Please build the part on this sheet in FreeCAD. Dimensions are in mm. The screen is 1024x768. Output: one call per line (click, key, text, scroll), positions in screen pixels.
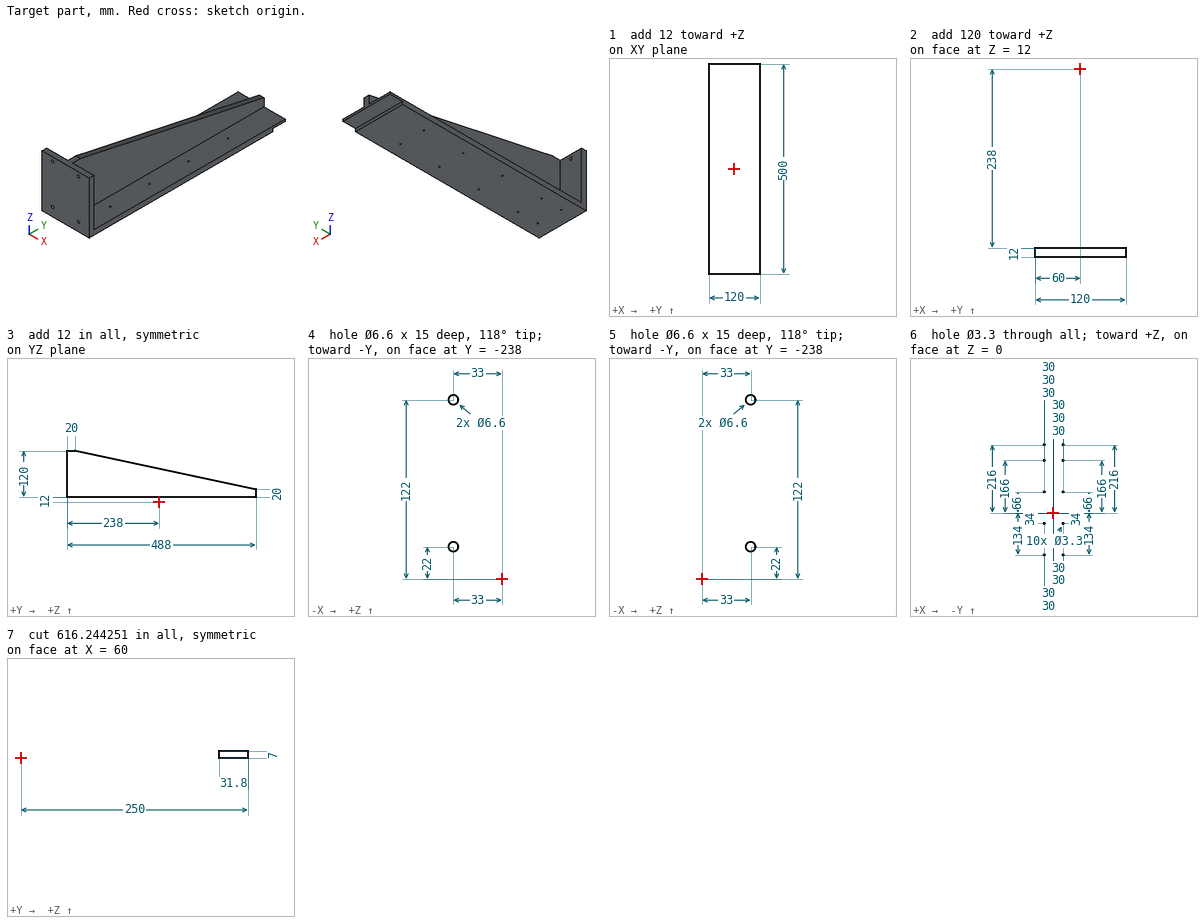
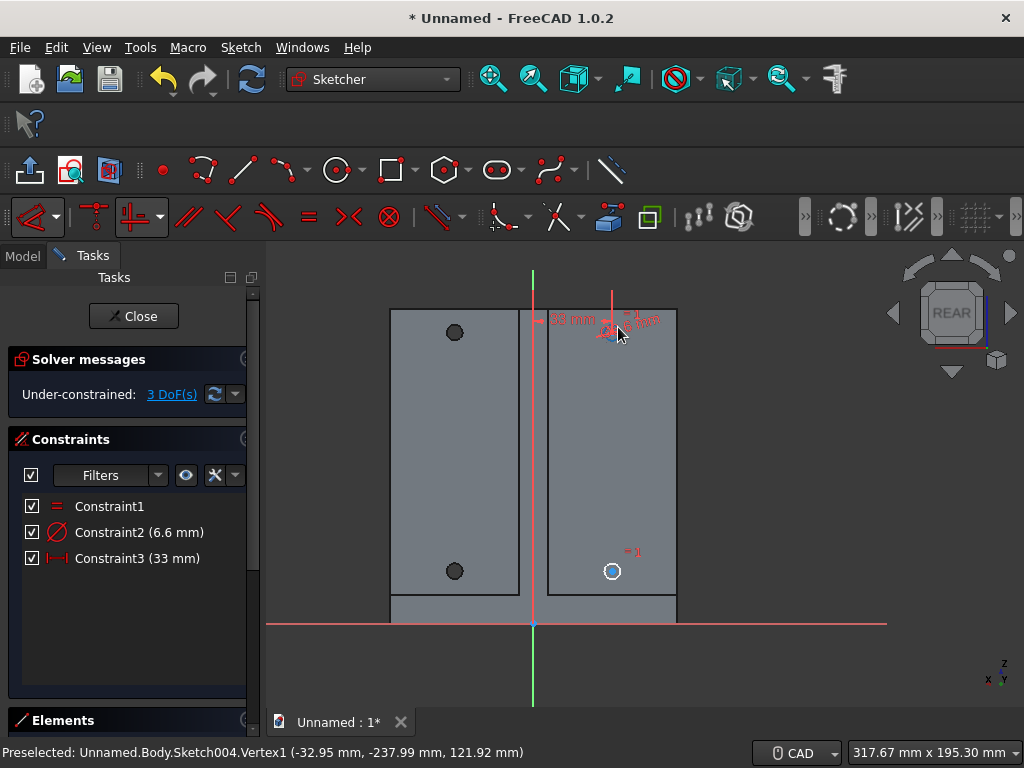
click(612, 571)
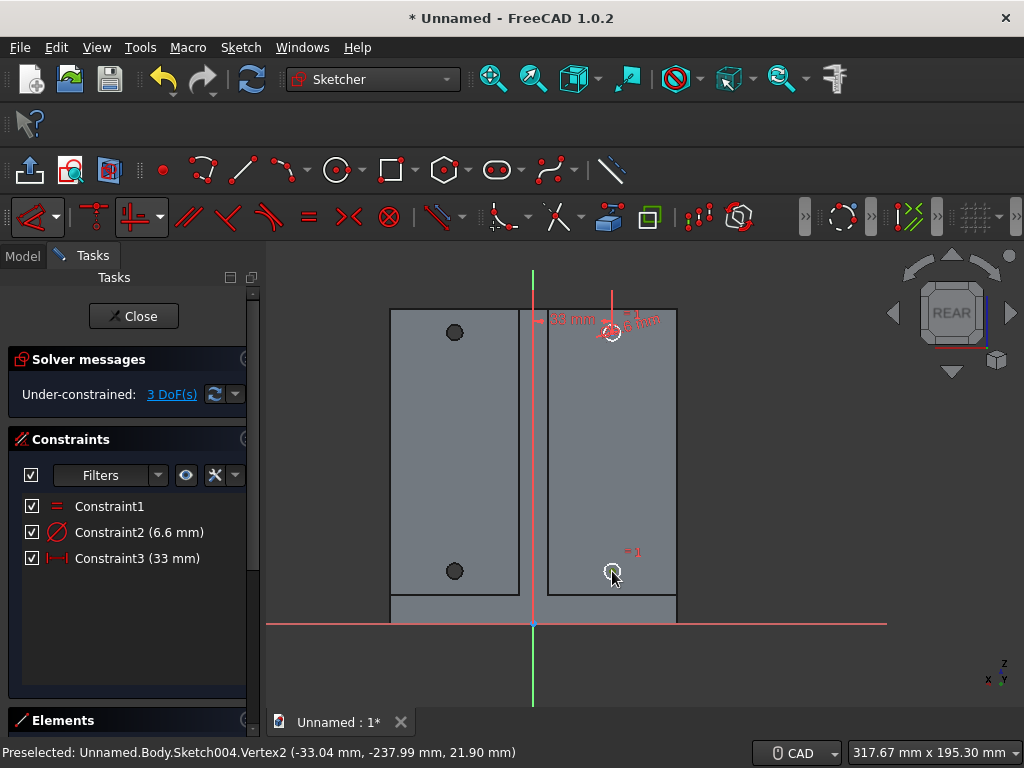
click(58, 218)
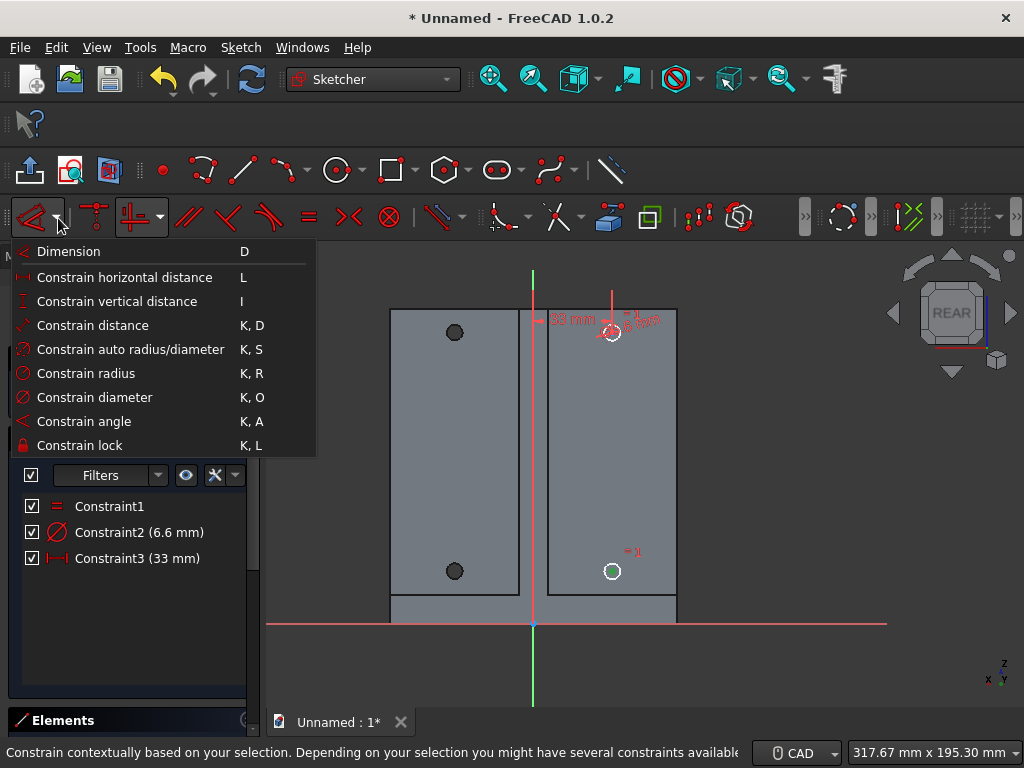
click(164, 277)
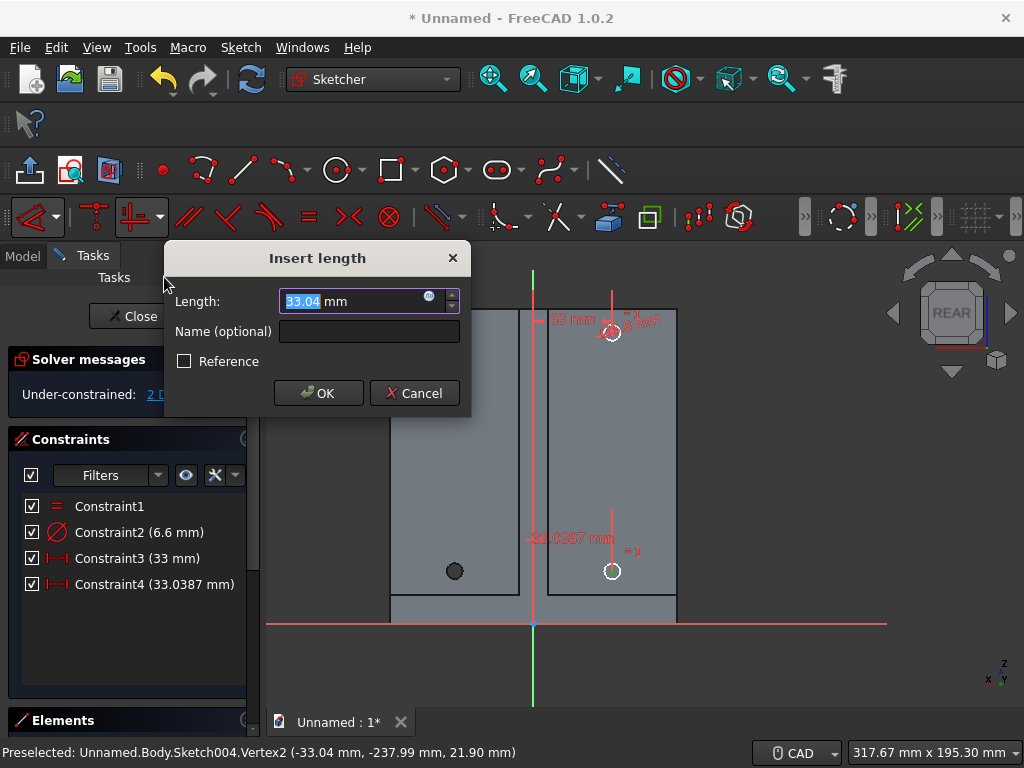
text(33)
key(Return)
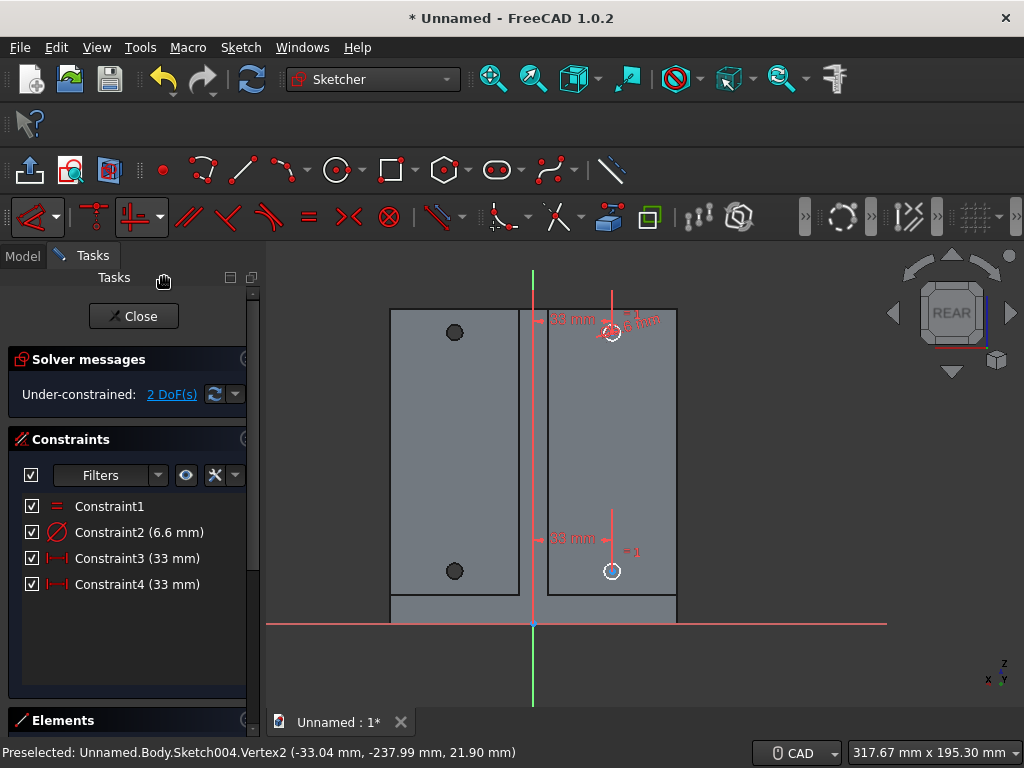
click(612, 571)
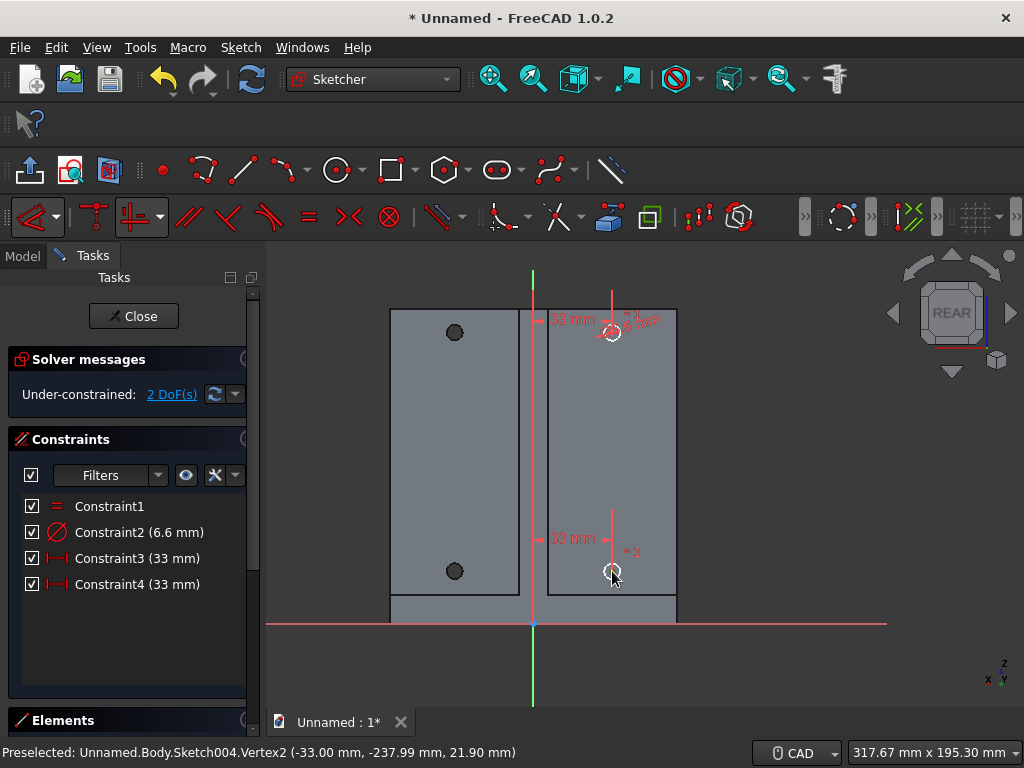
click(58, 218)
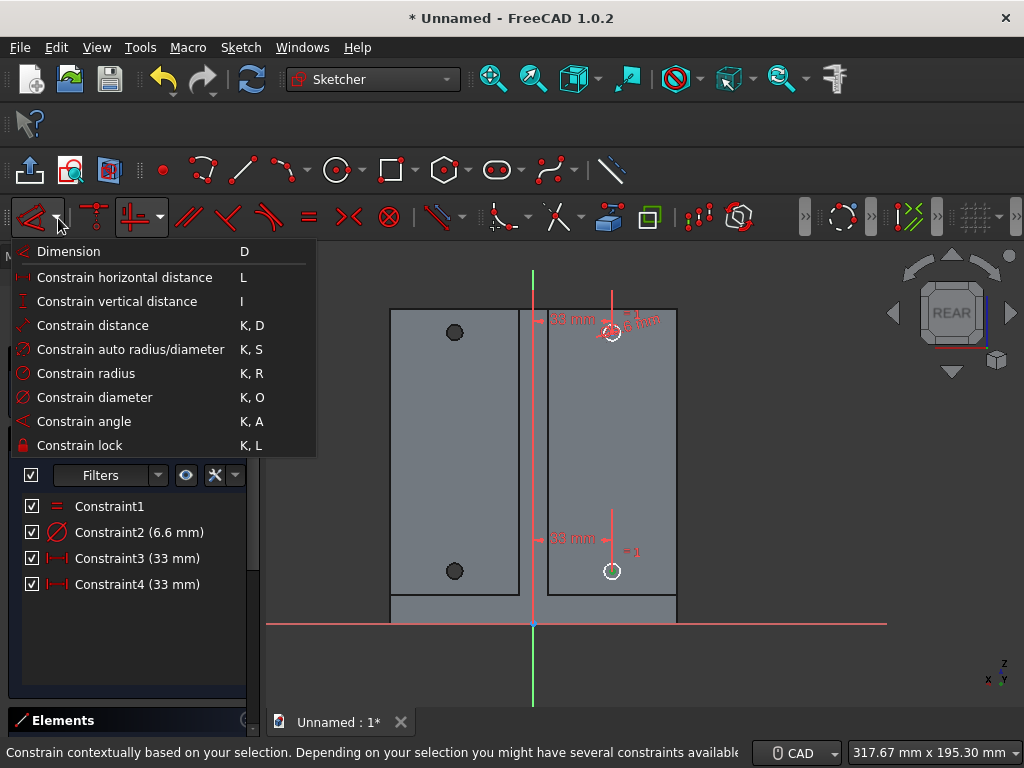
click(164, 301)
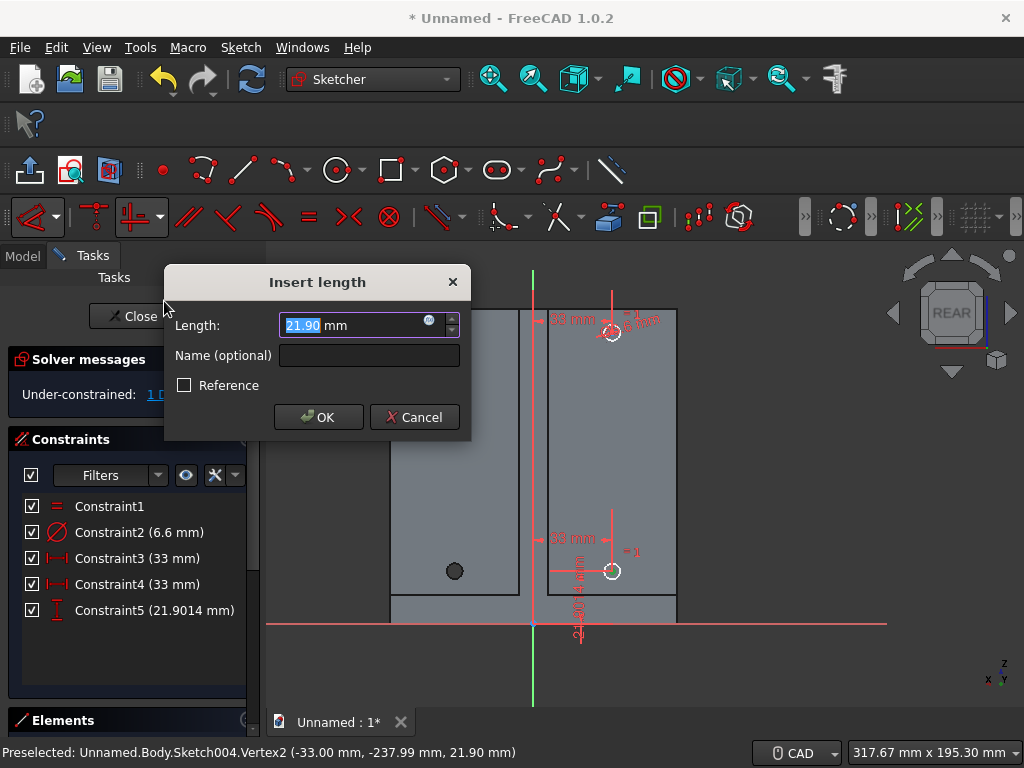
text(22)
key(Return)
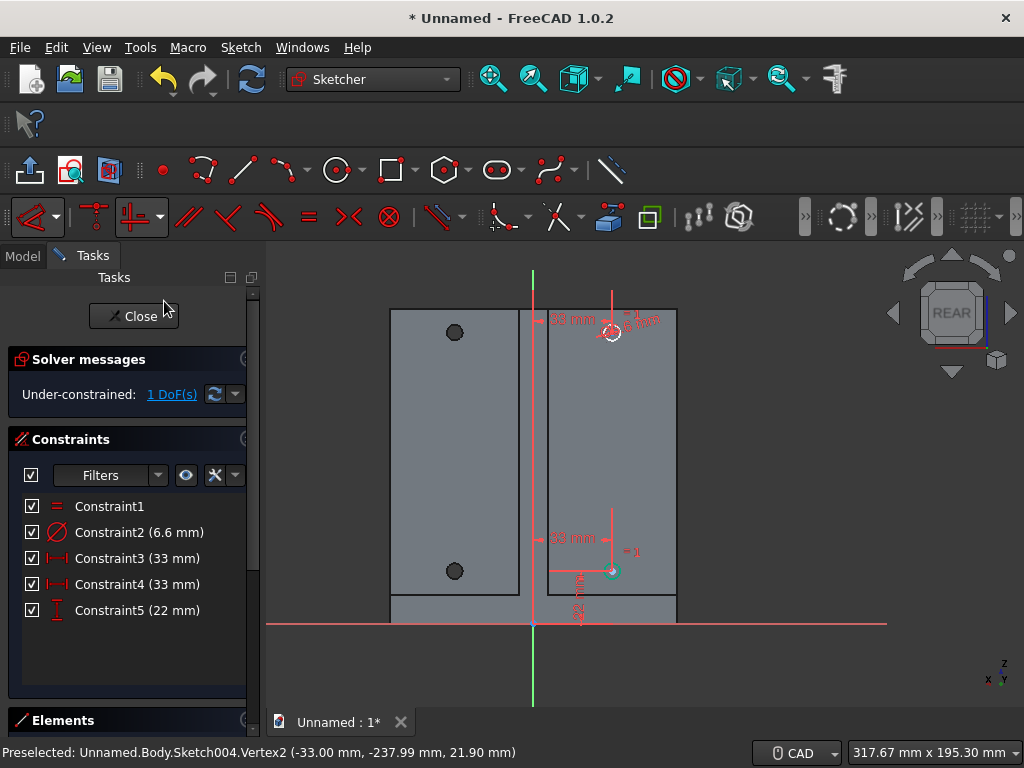
click(612, 333)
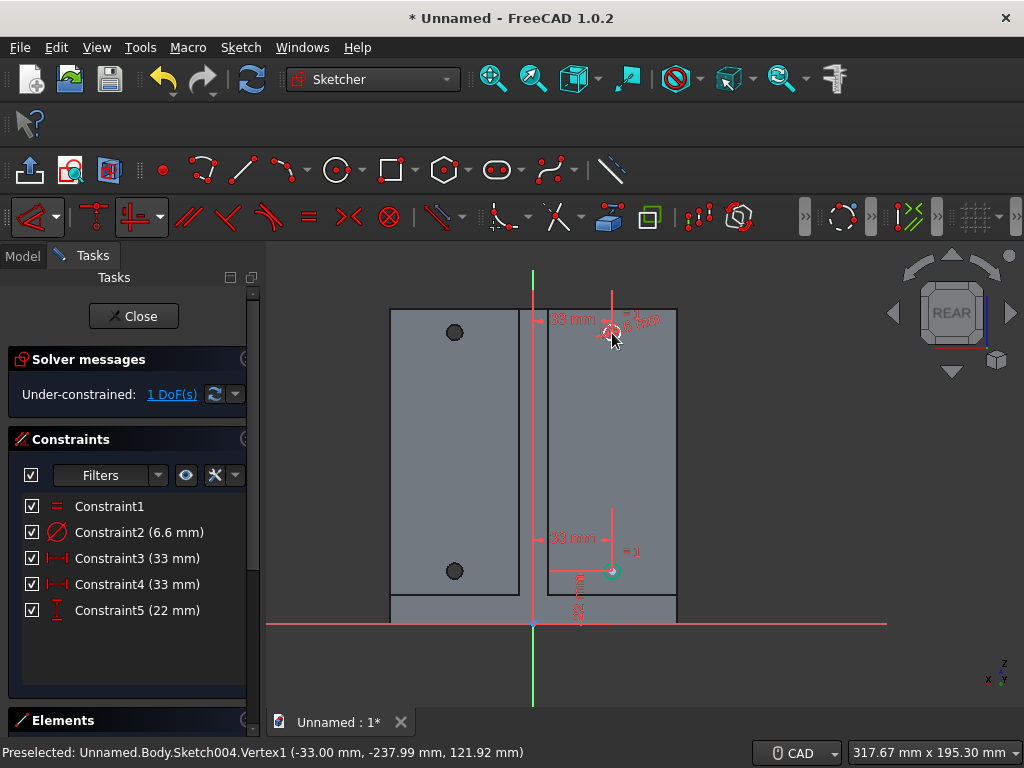
click(58, 218)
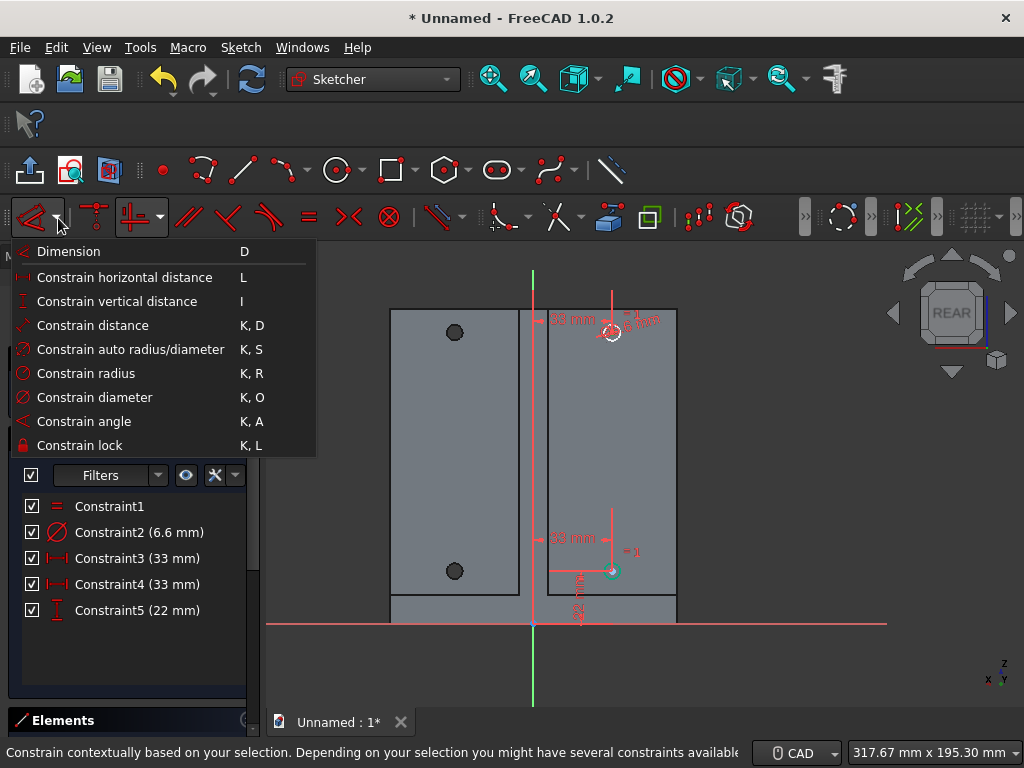
click(164, 301)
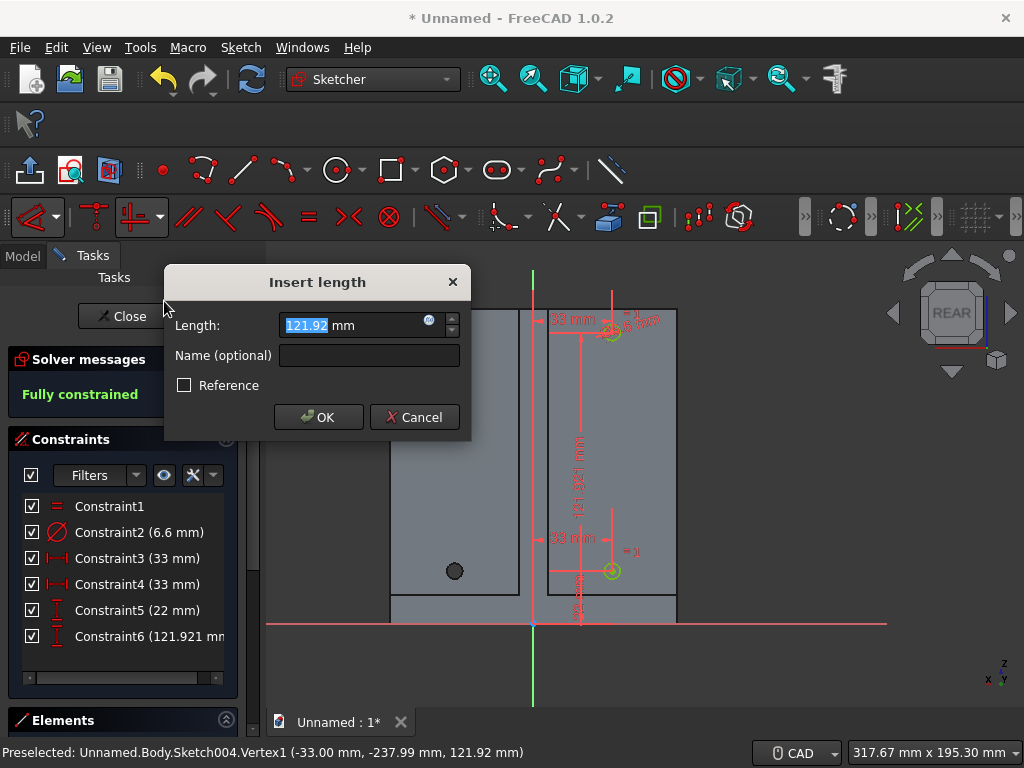
text(122)
key(Return)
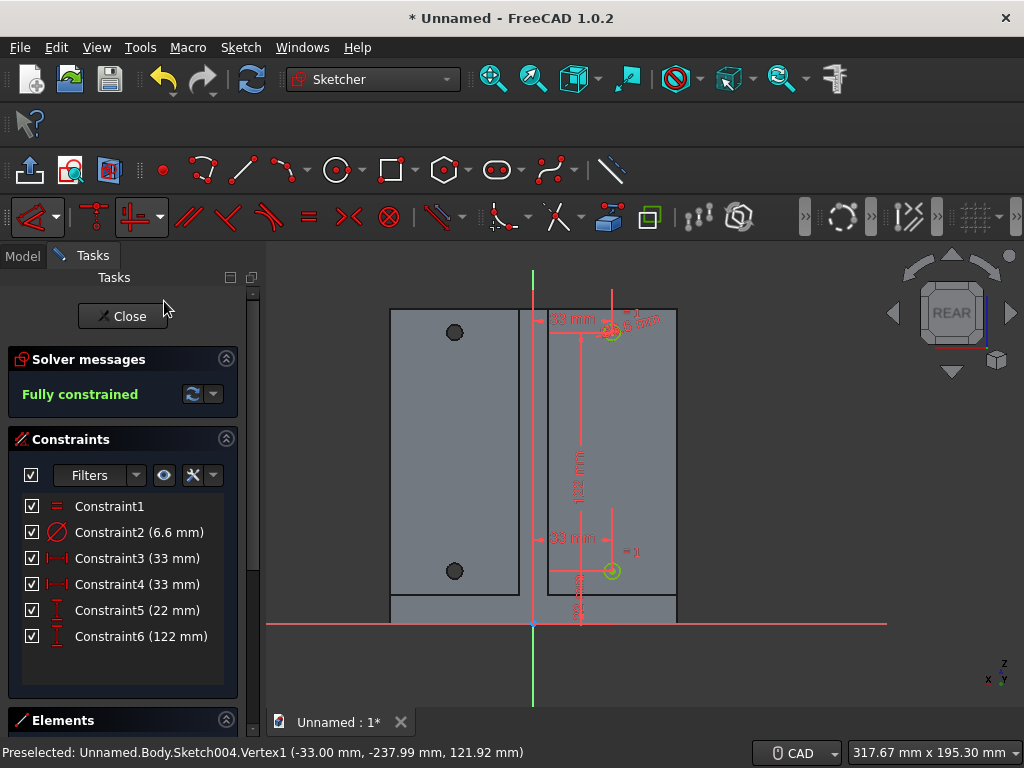
click(123, 316)